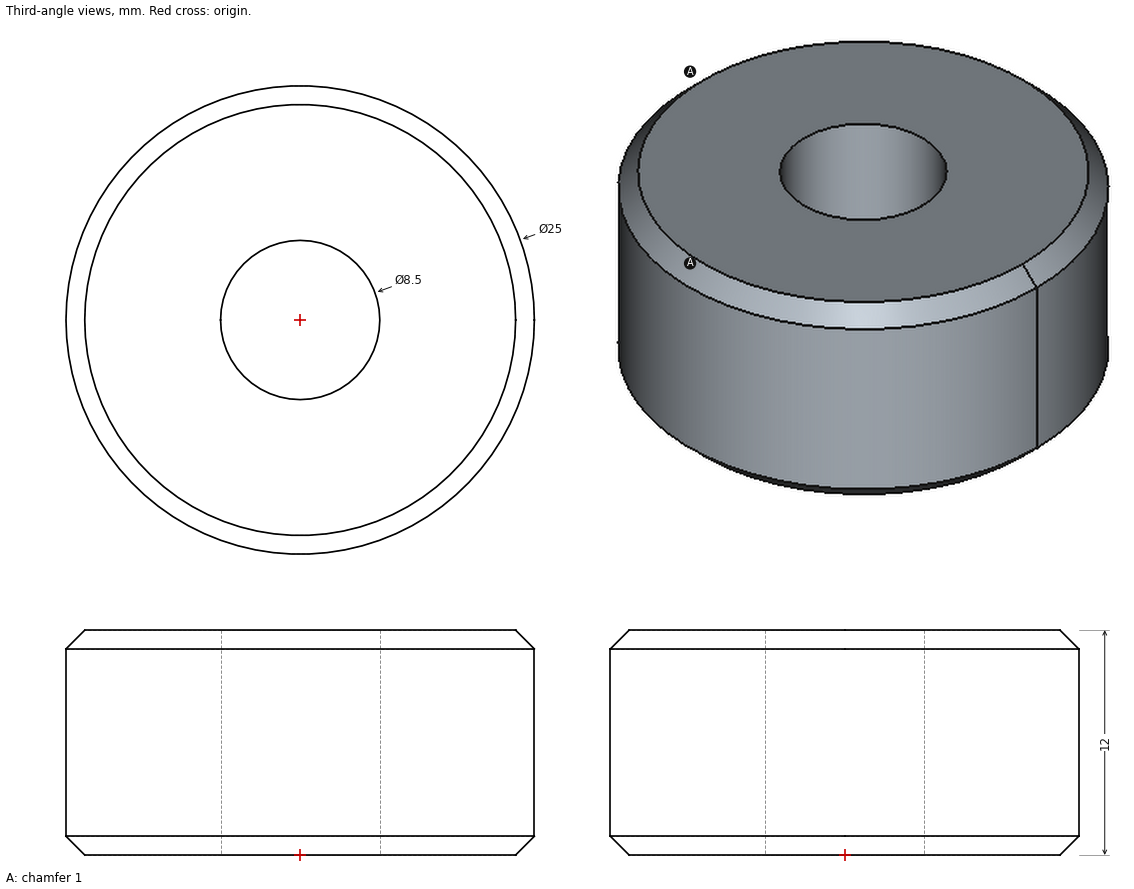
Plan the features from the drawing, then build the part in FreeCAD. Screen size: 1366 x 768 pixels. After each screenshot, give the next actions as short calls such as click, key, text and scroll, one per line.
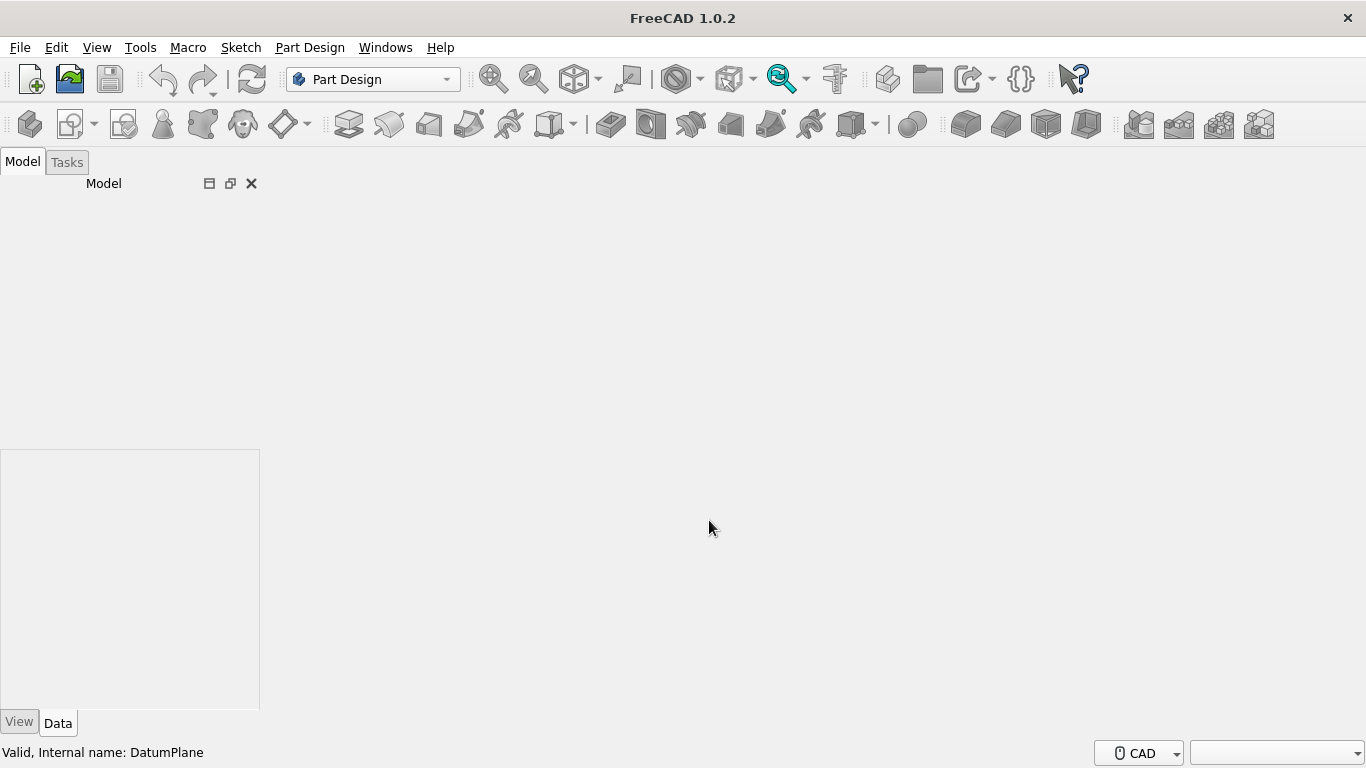
click(30, 80)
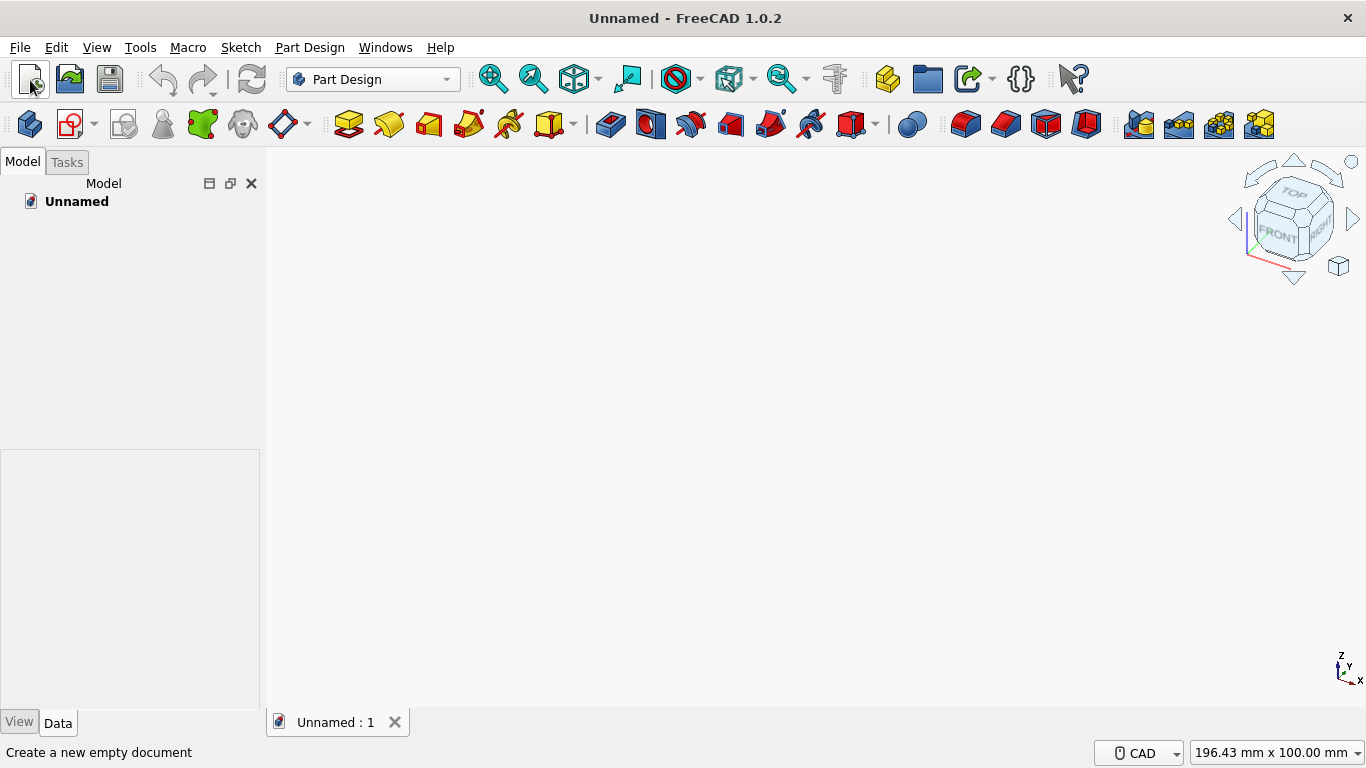
click(70, 124)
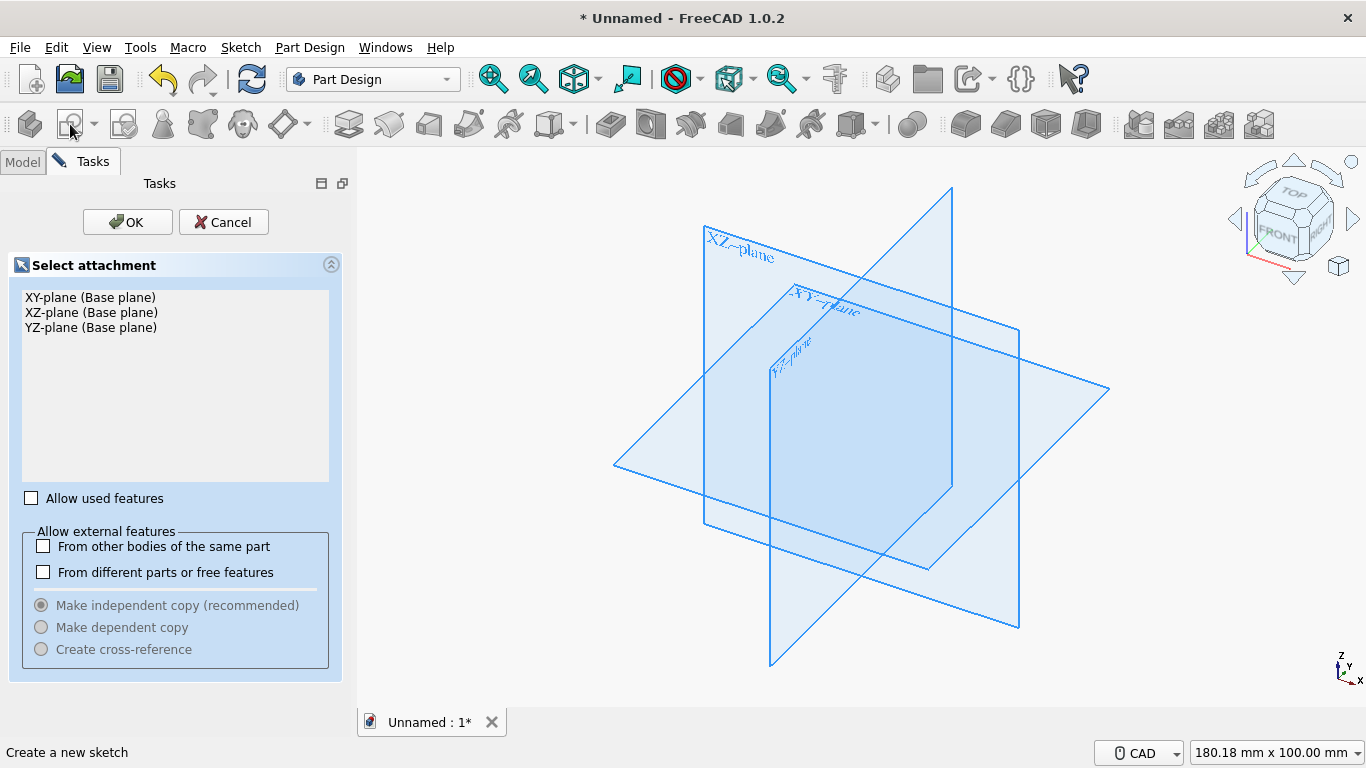
click(82, 298)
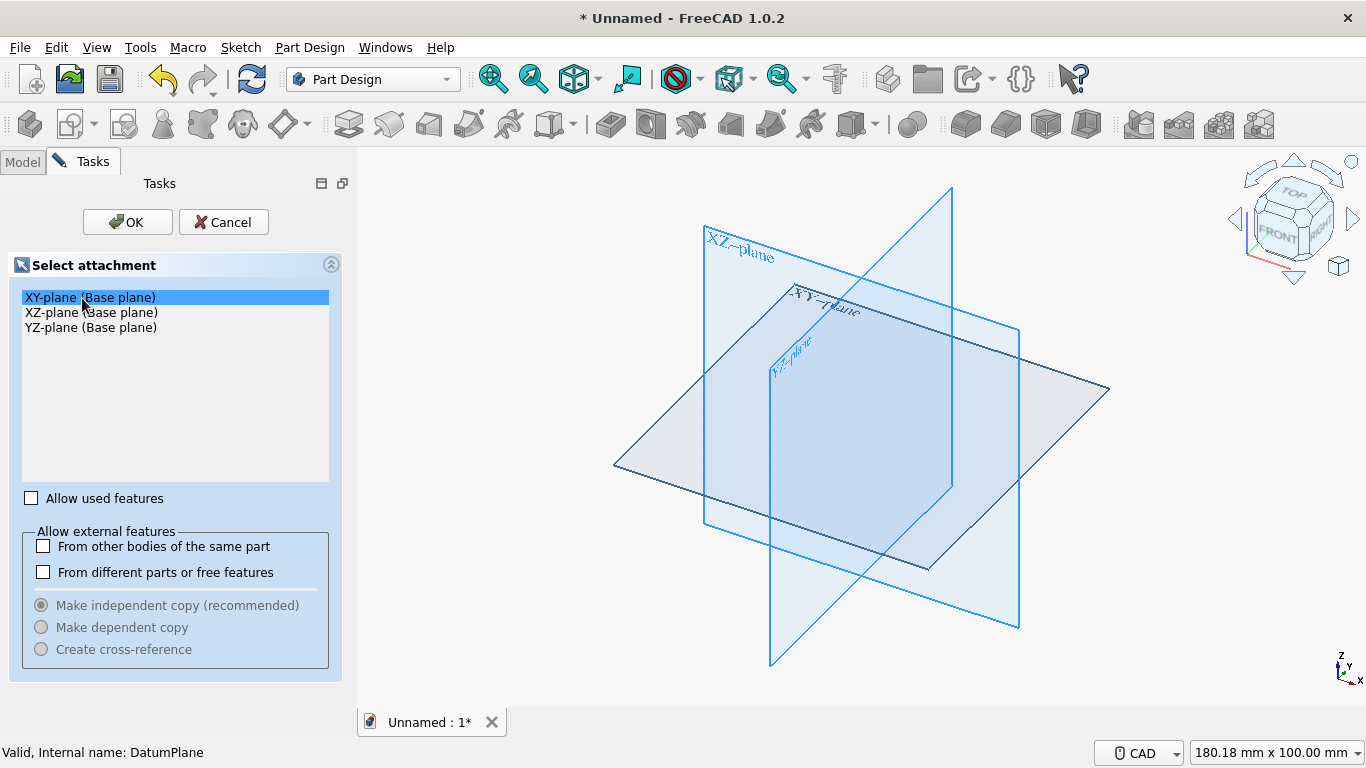
click(128, 222)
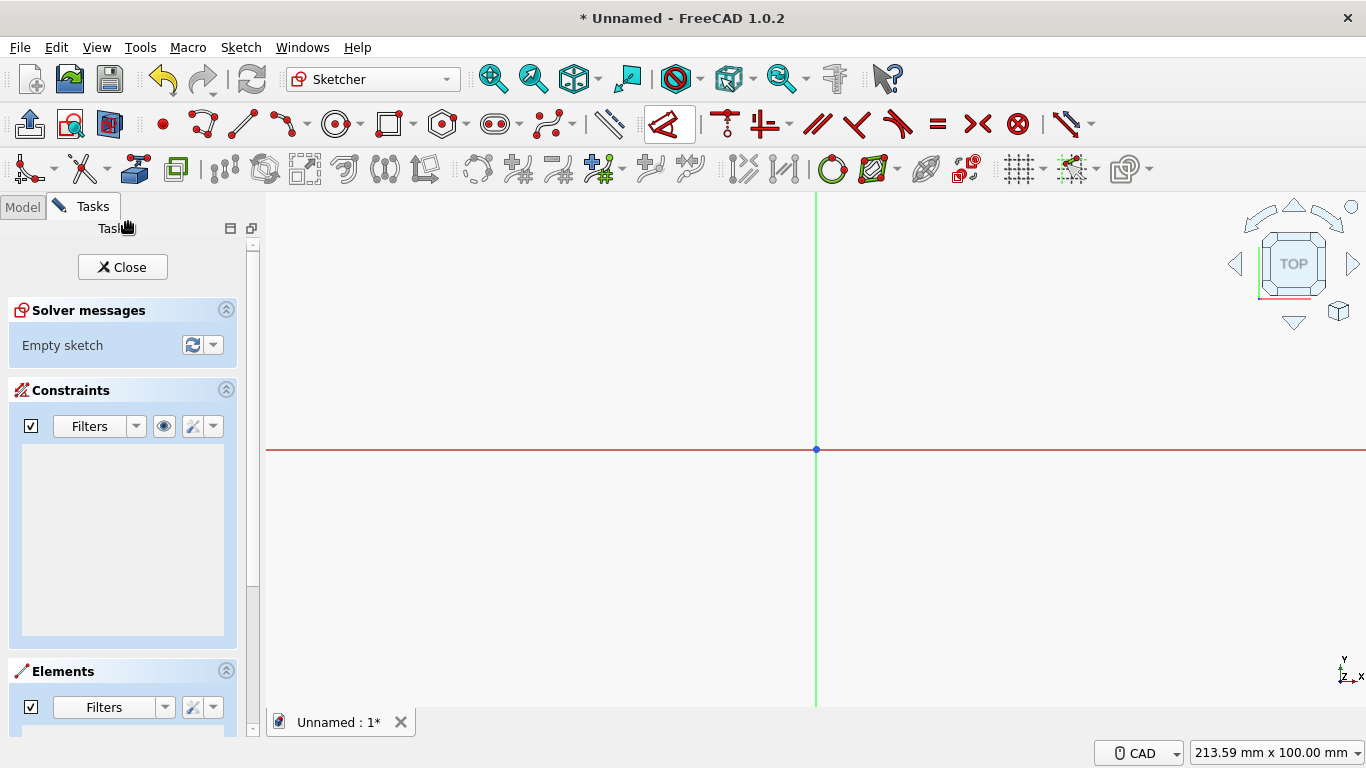
scroll(856, 449, up, 5)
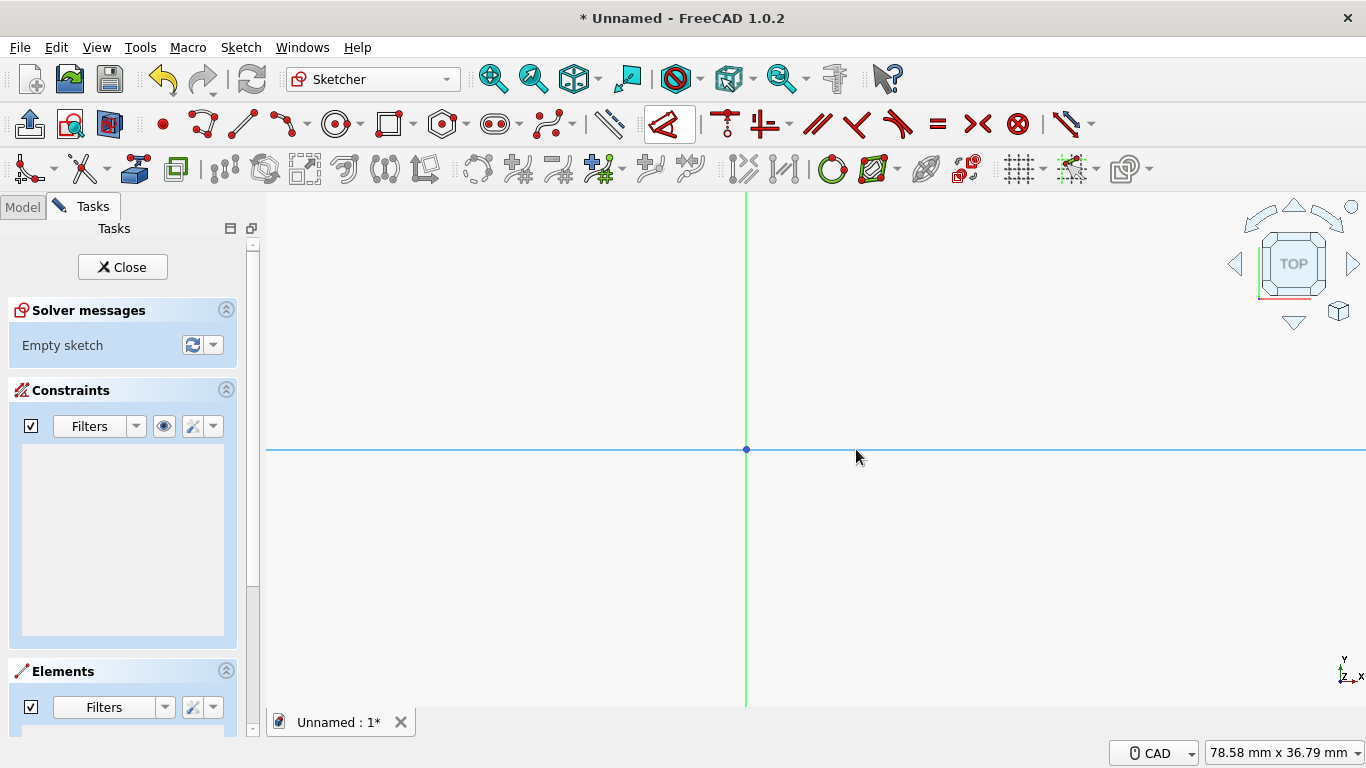
click(336, 124)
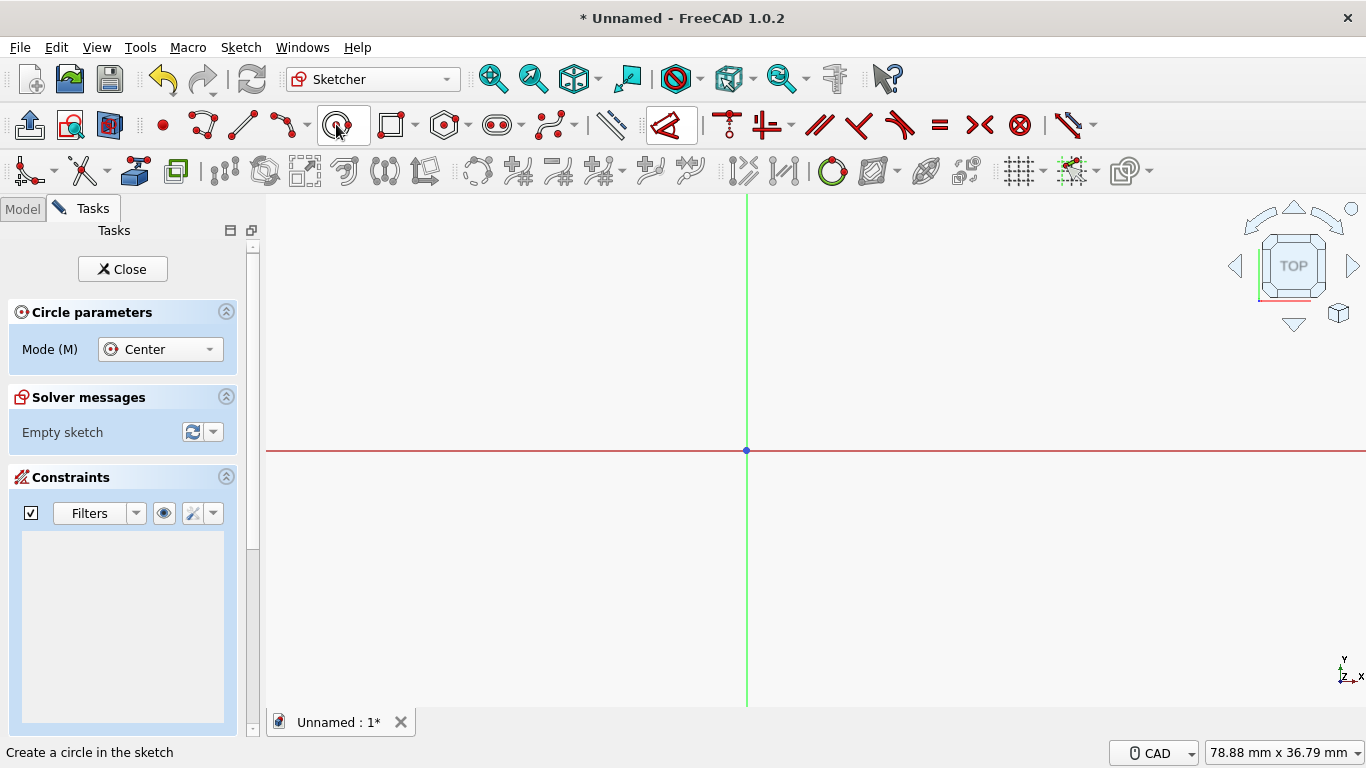
click(747, 450)
click(870, 327)
key(Escape)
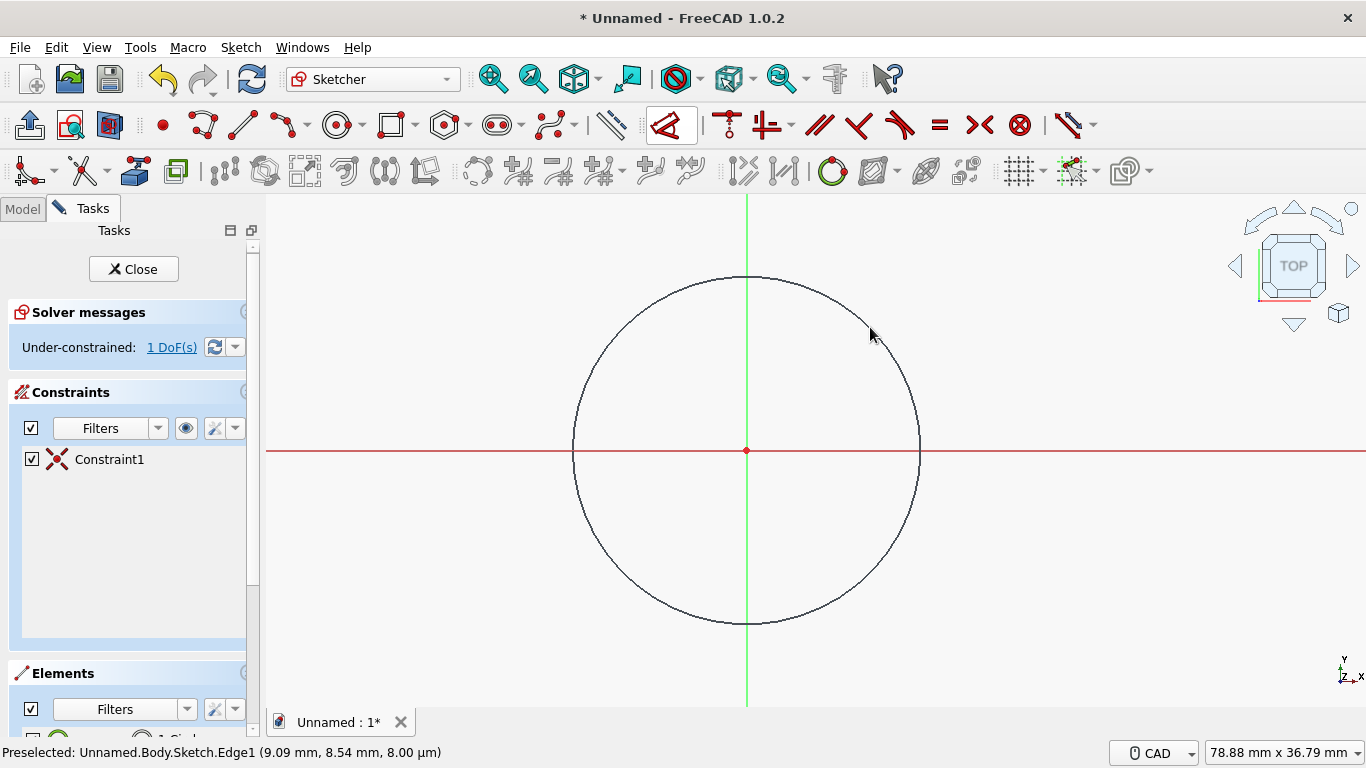
key(d)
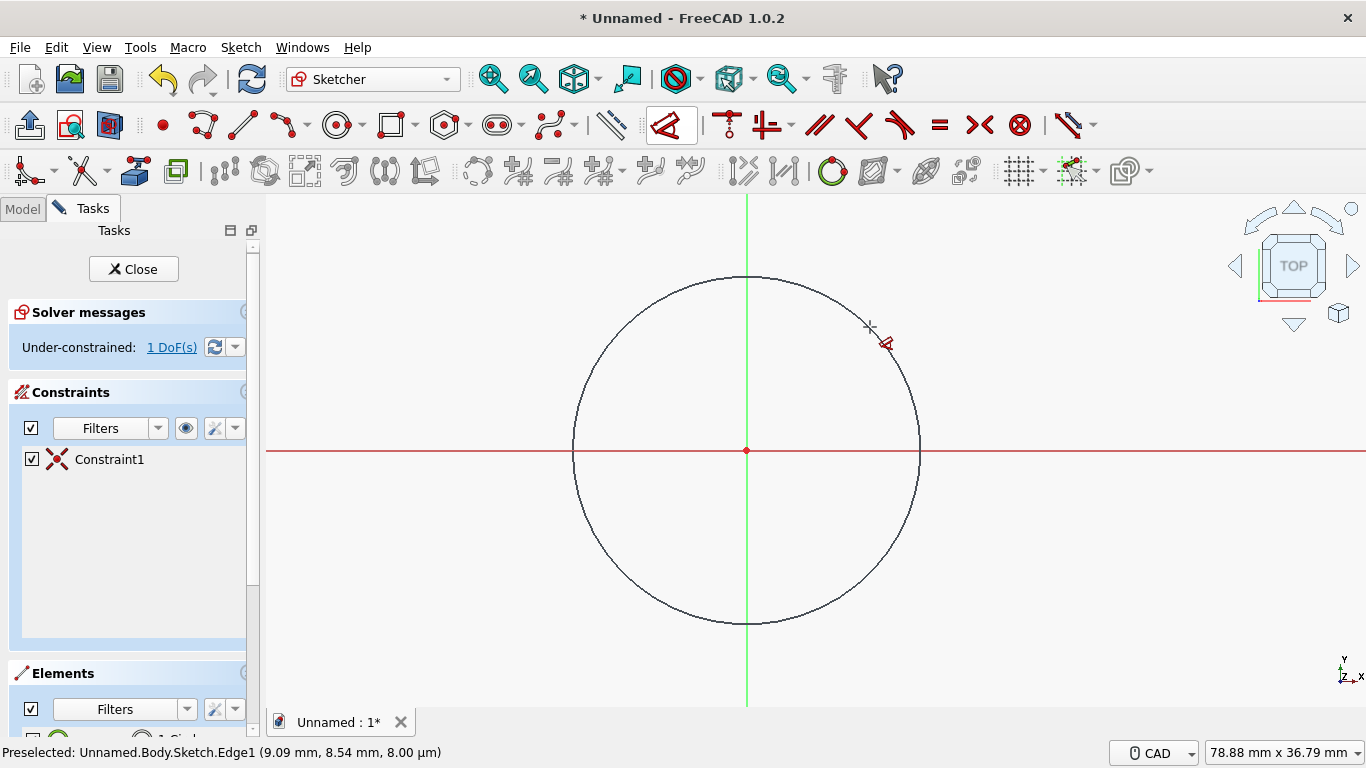
click(869, 327)
click(892, 304)